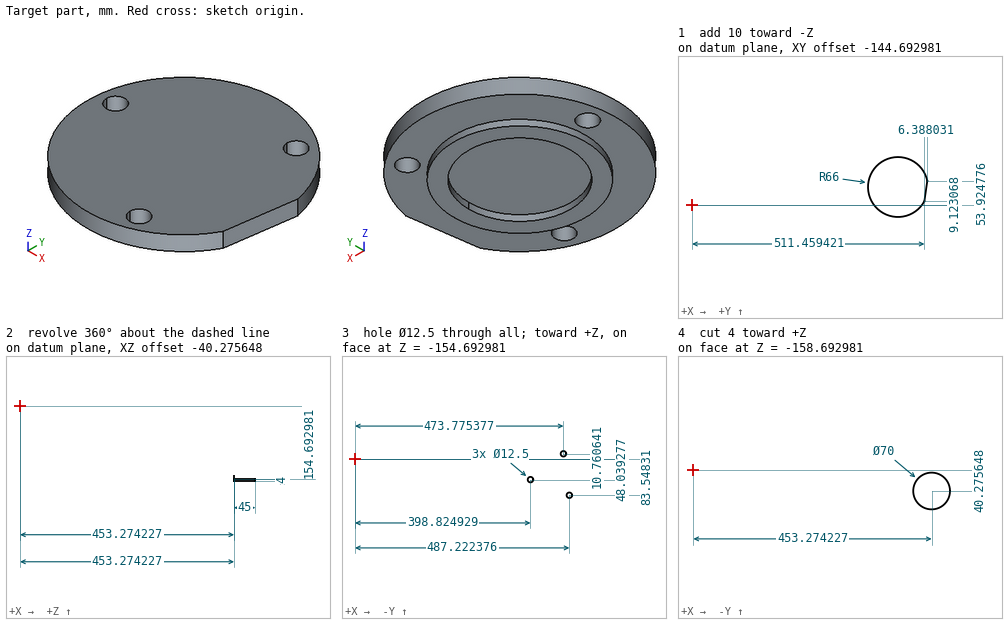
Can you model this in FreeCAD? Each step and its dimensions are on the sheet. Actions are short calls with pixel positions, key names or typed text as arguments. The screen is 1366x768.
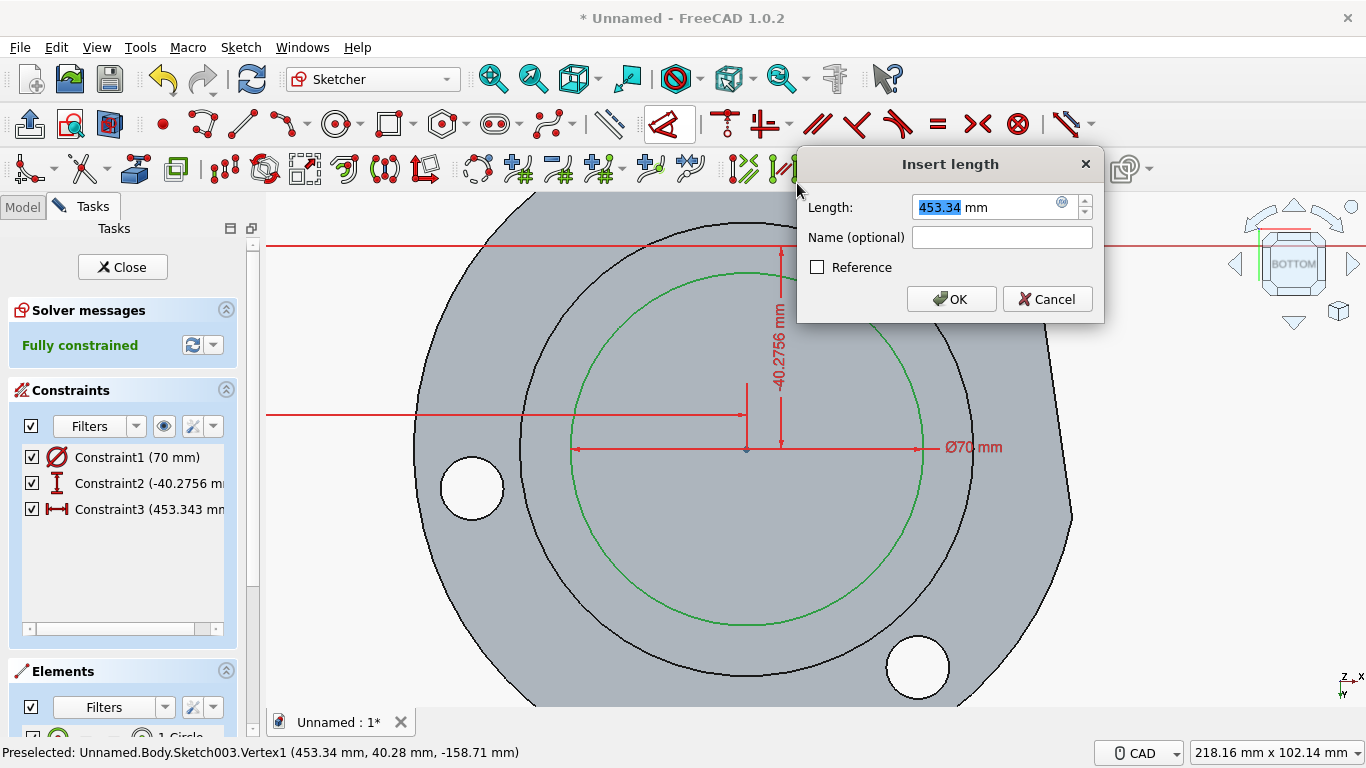
text(453.274227)
key(Return)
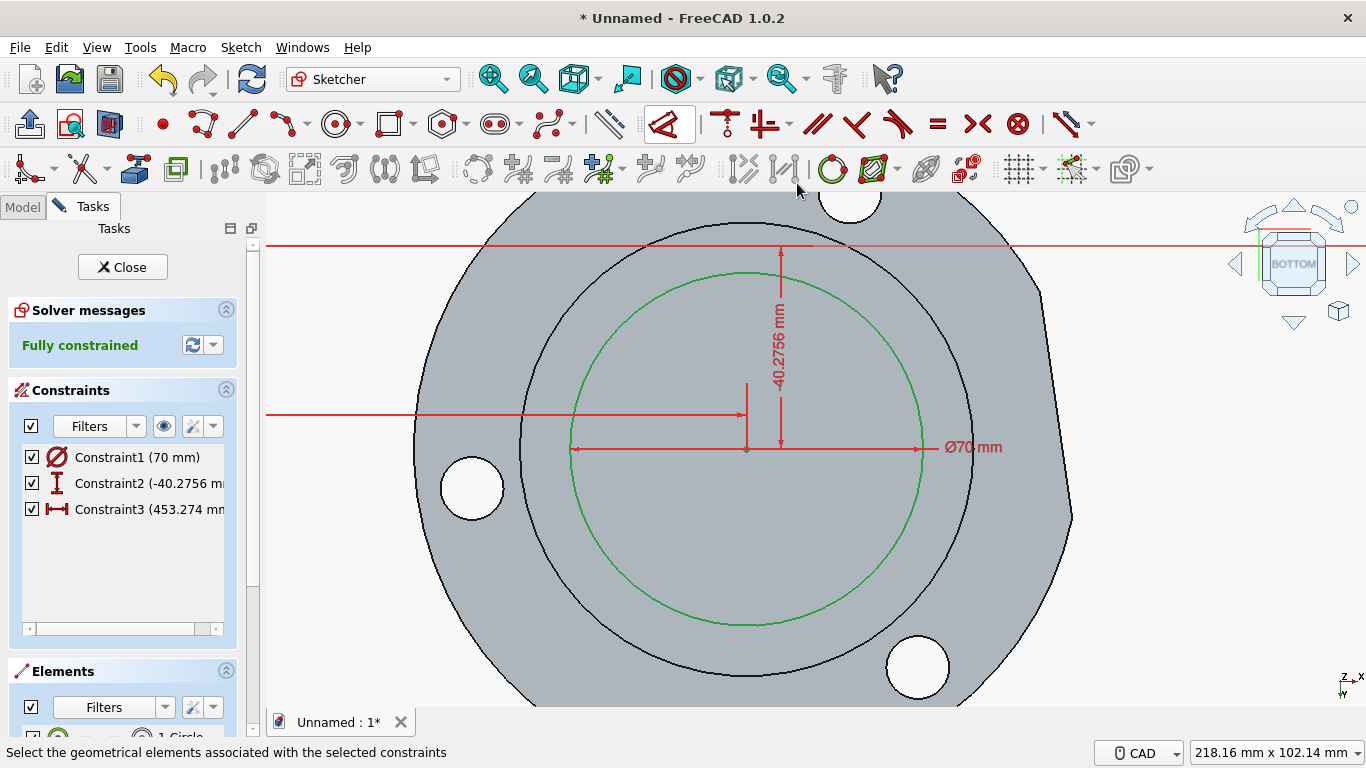
click(123, 267)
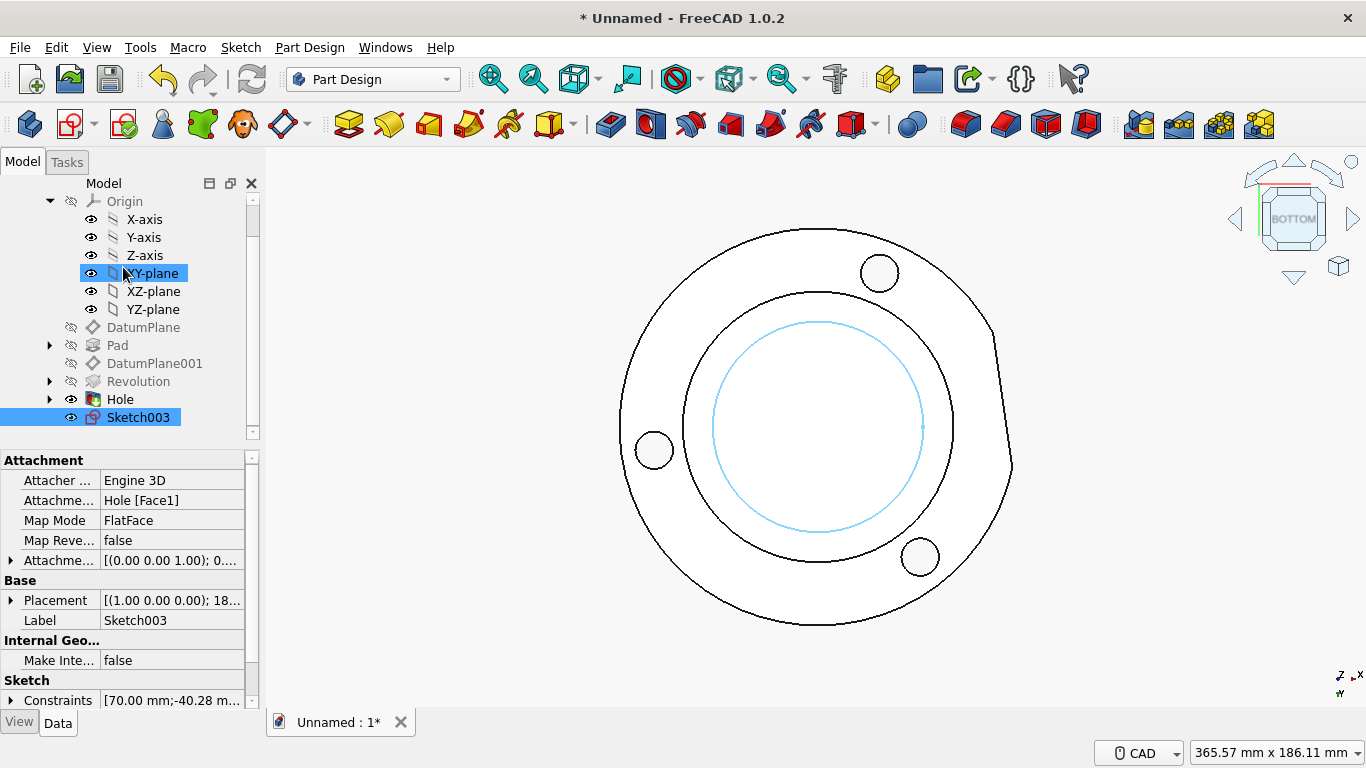
click(612, 124)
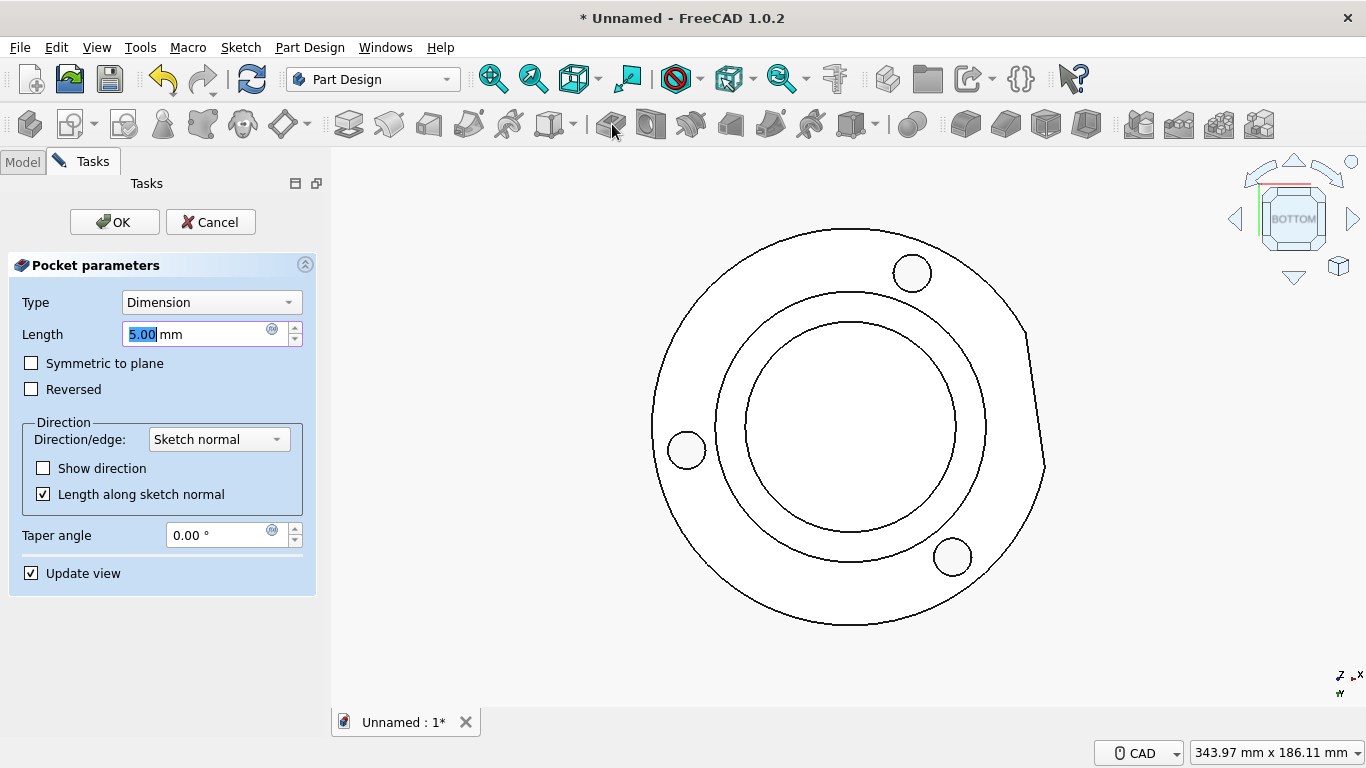
text(4)
key(Tab)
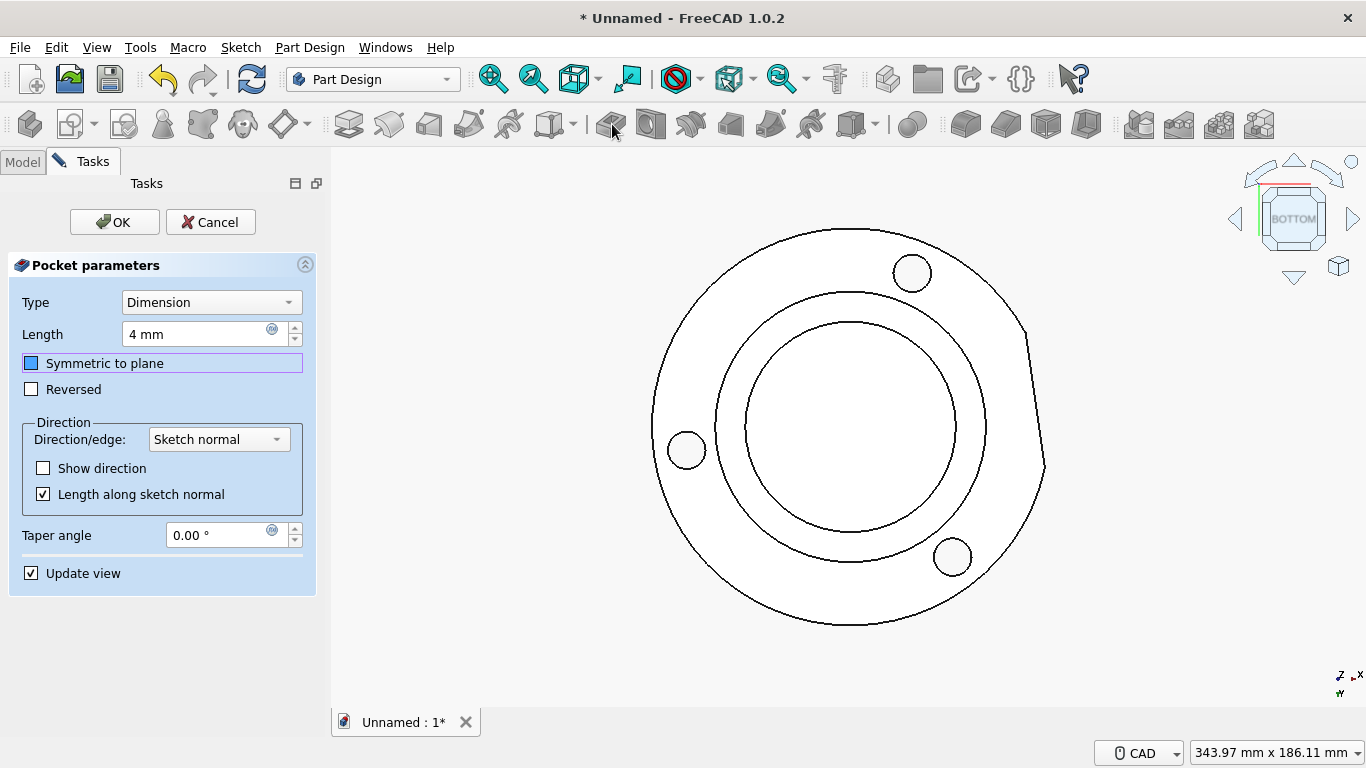
click(115, 222)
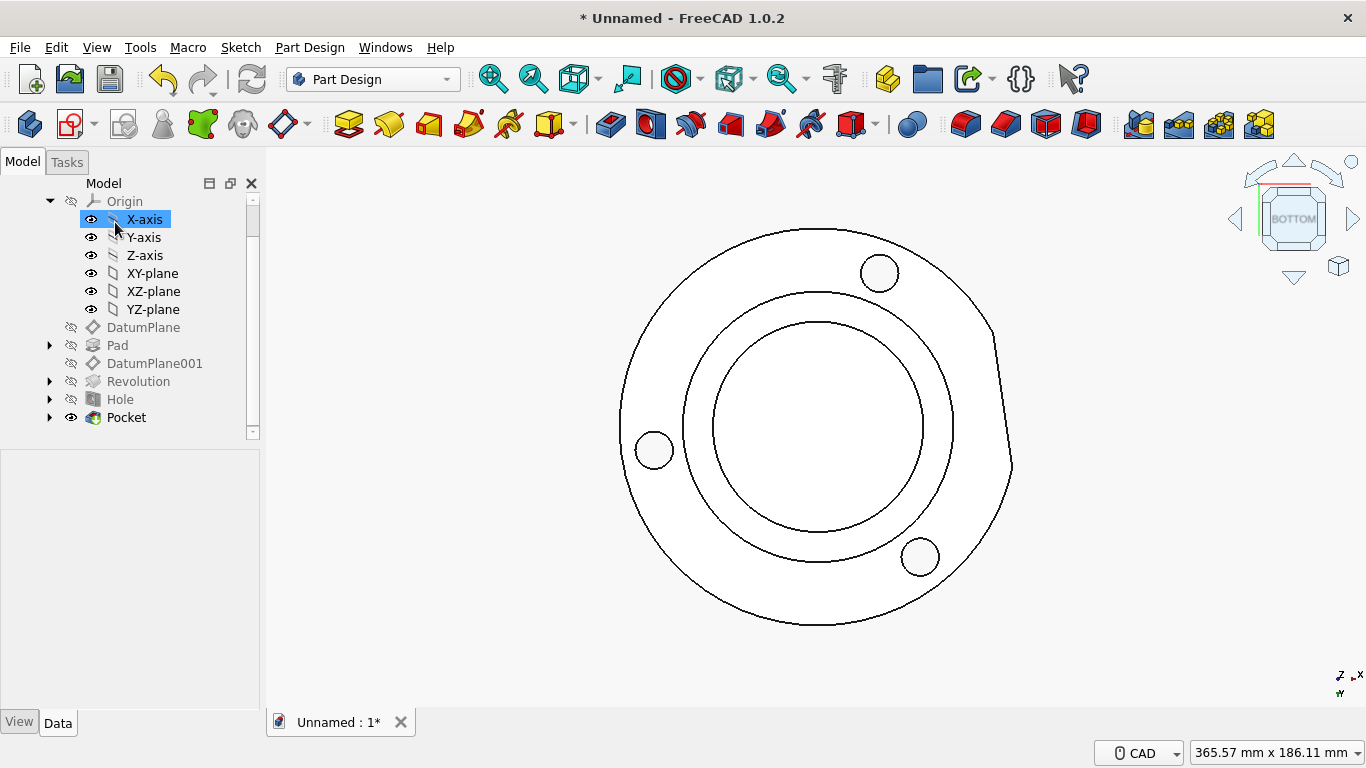
key(0)